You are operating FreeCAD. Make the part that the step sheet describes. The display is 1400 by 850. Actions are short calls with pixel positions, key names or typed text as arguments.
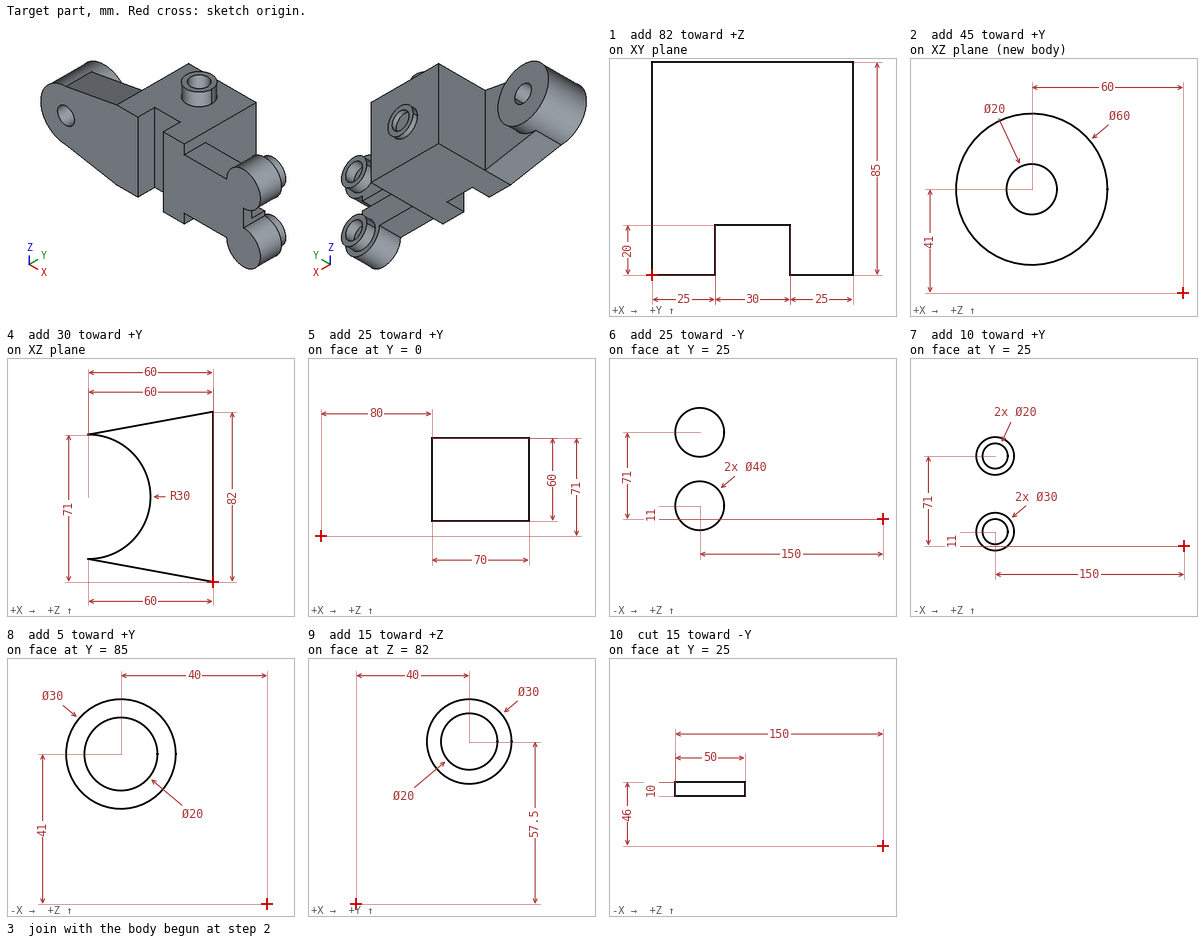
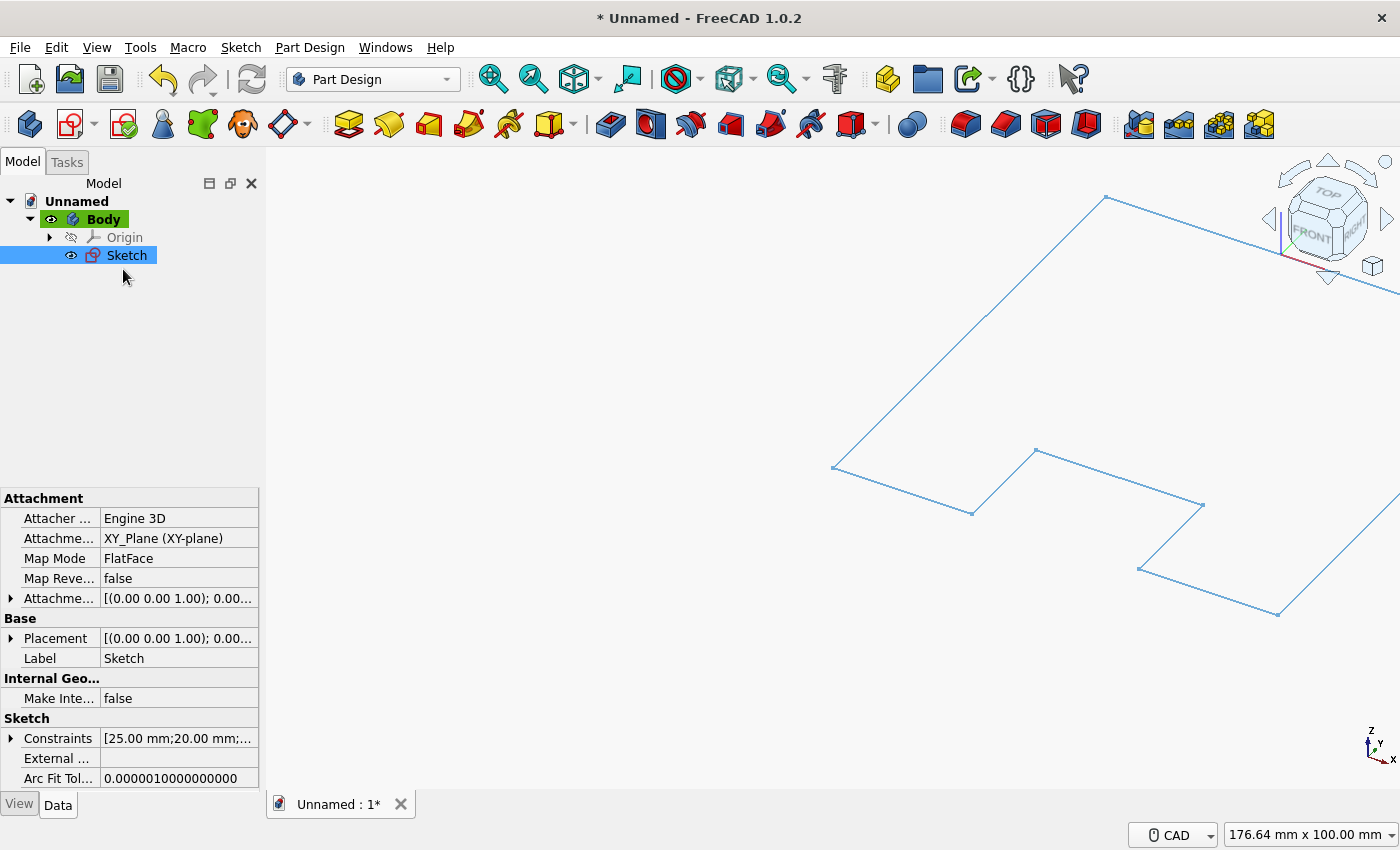
click(350, 124)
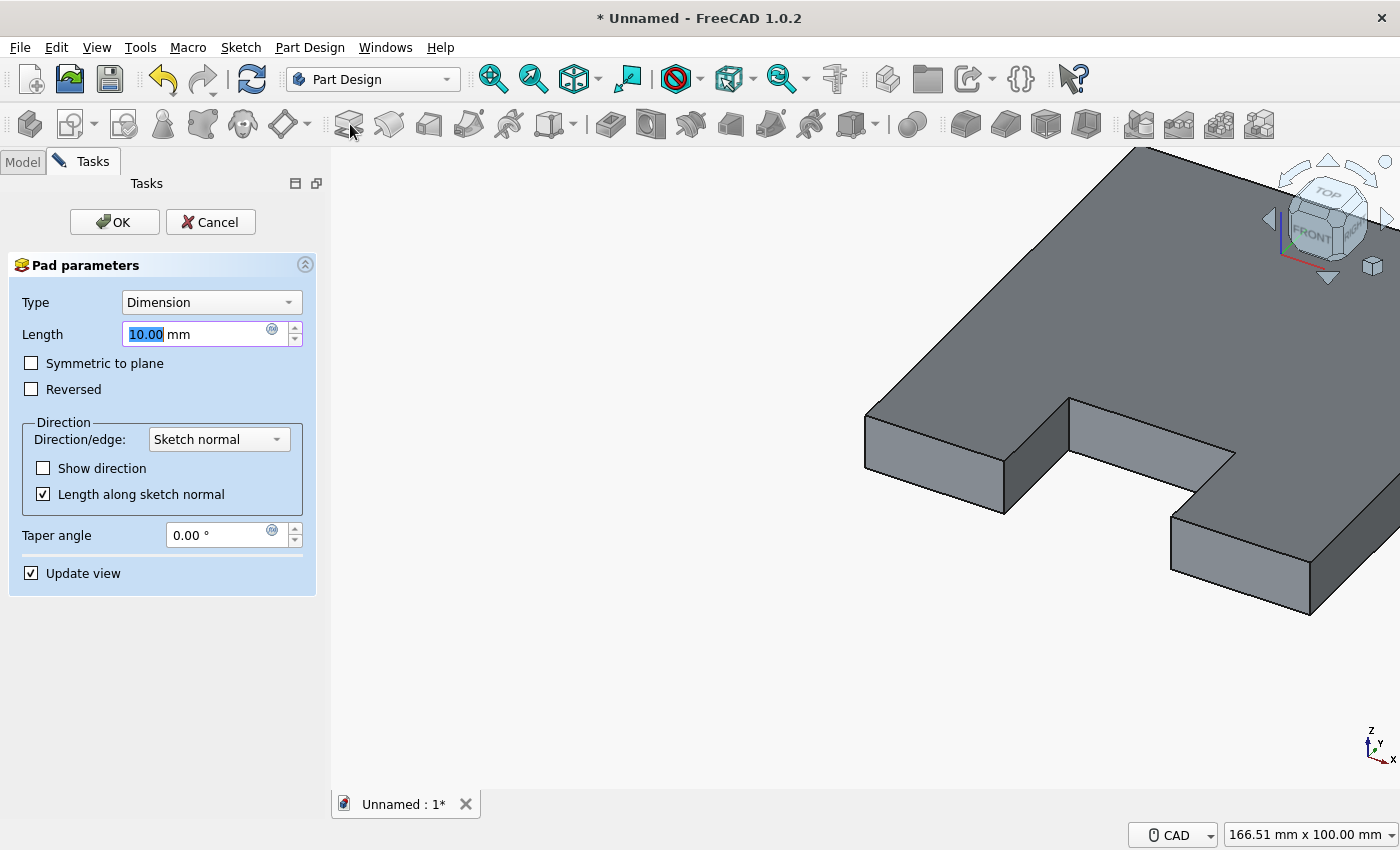
text(82)
key(Tab)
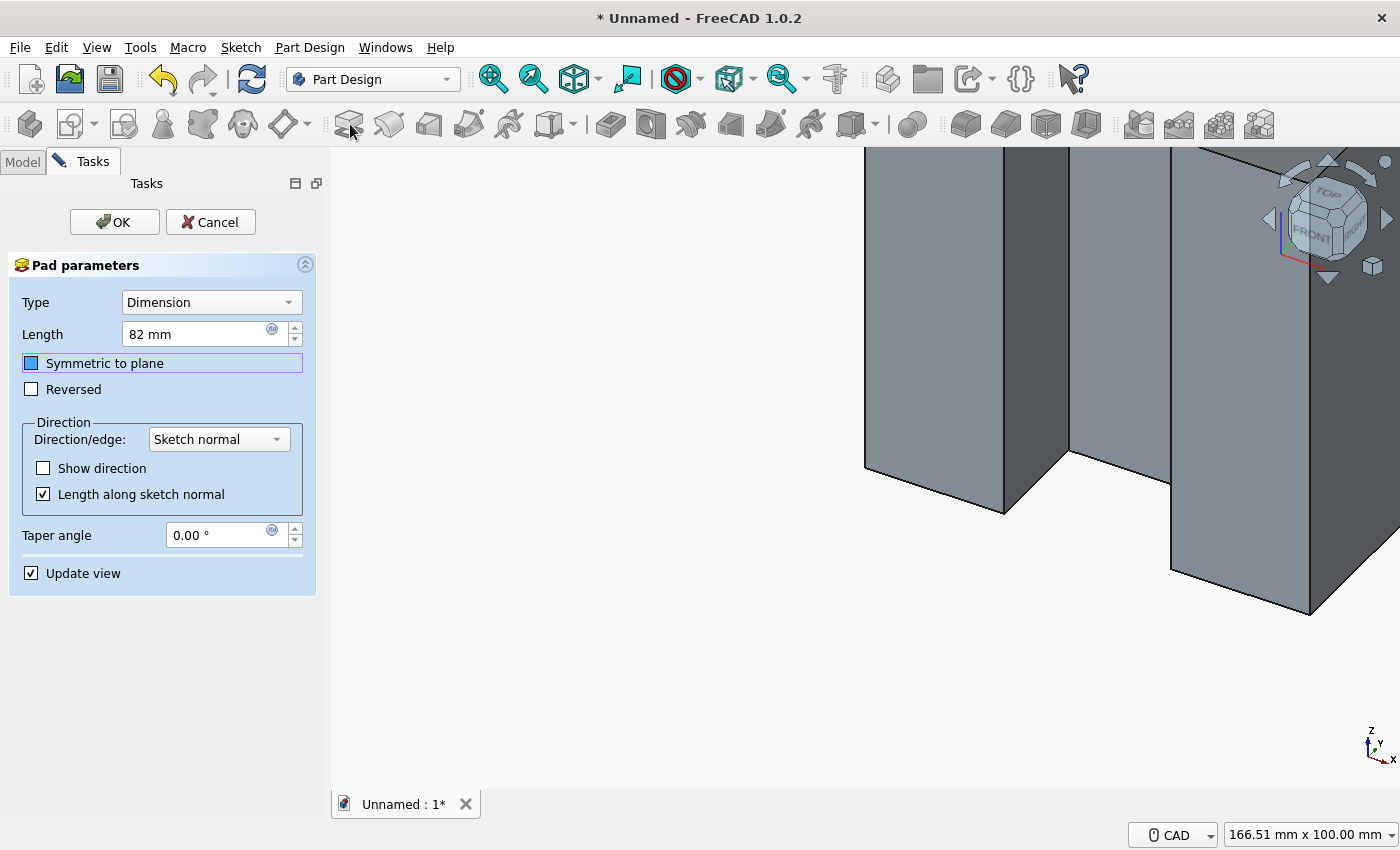
click(115, 222)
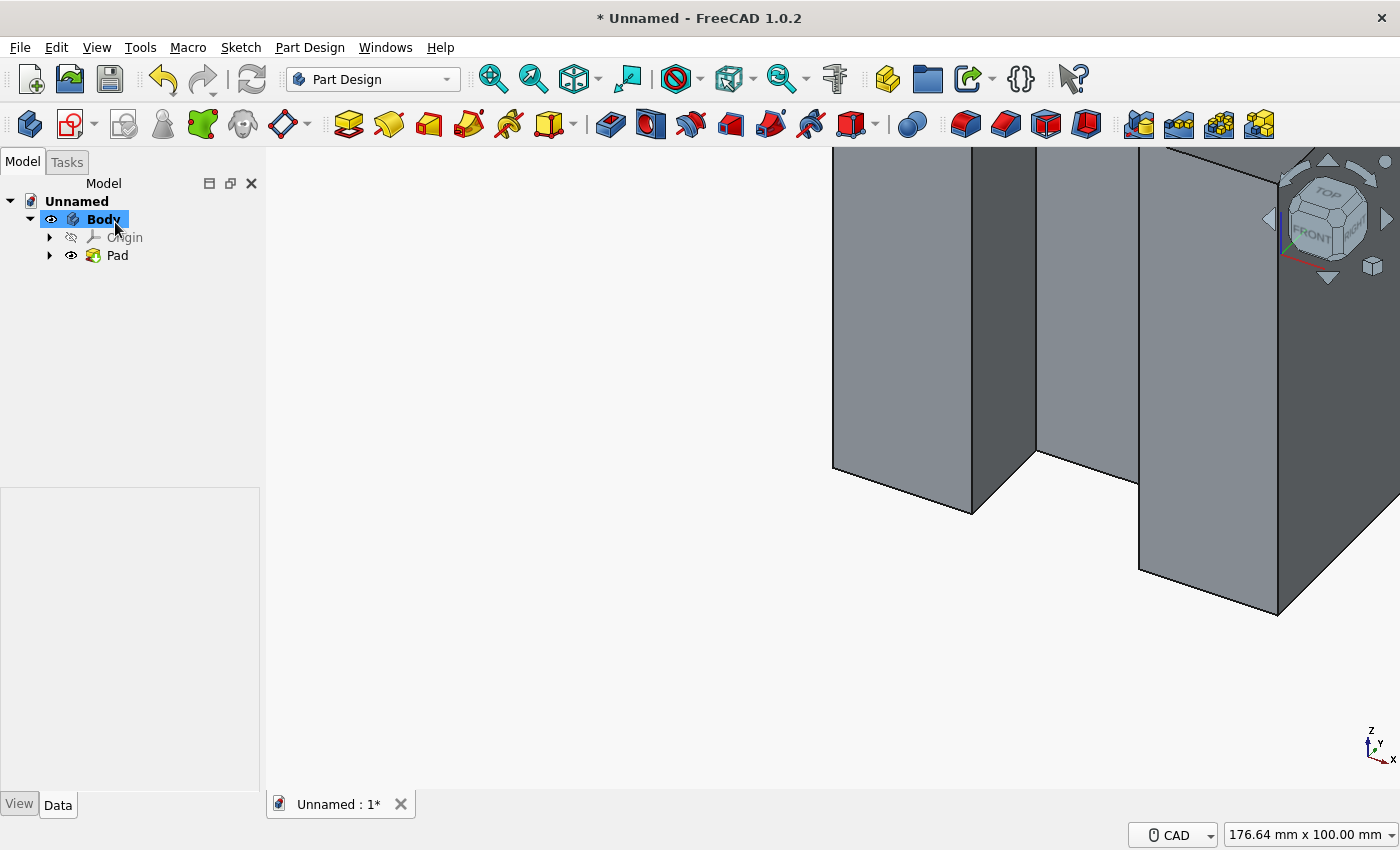
key(v)
key(f)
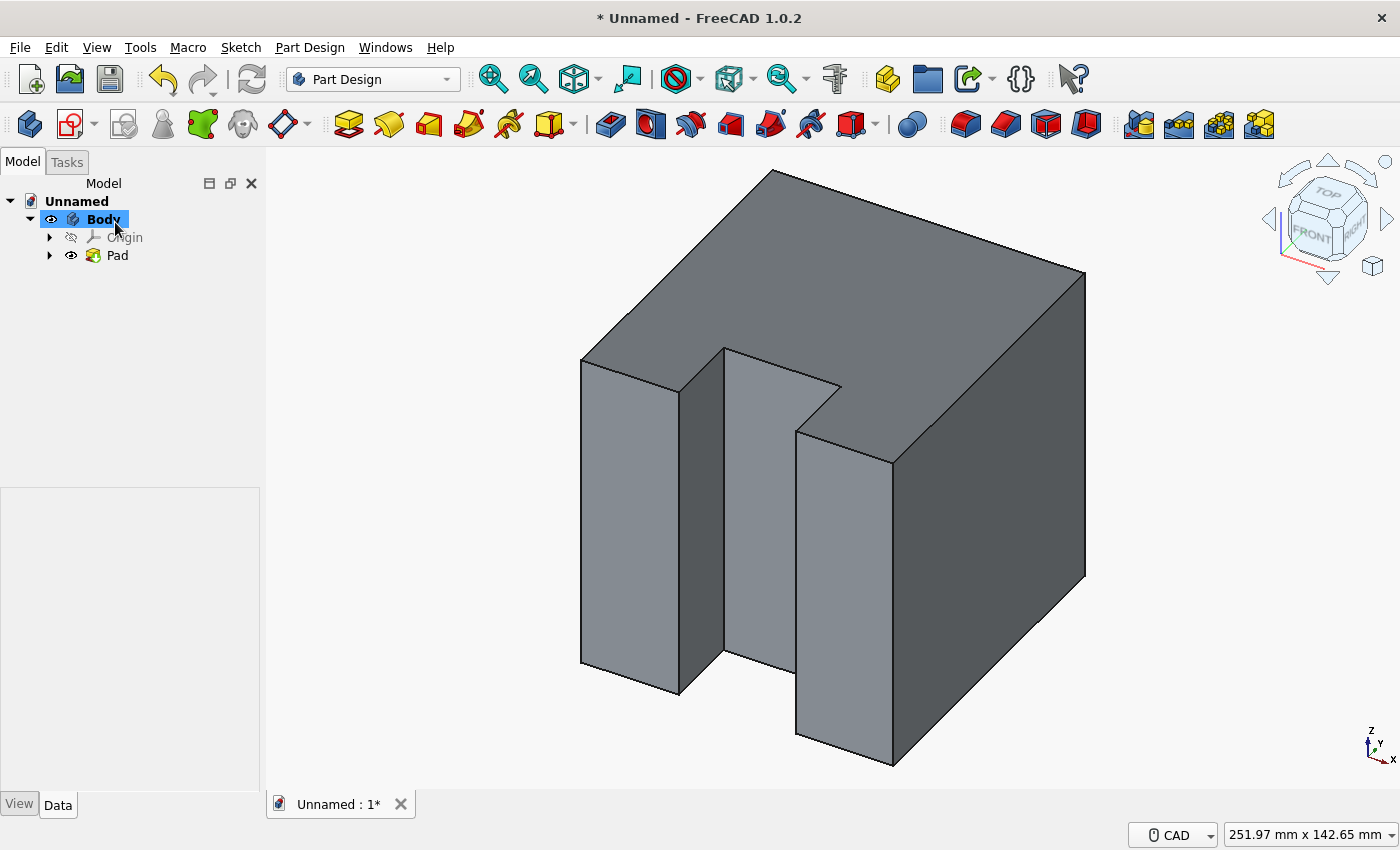
click(30, 124)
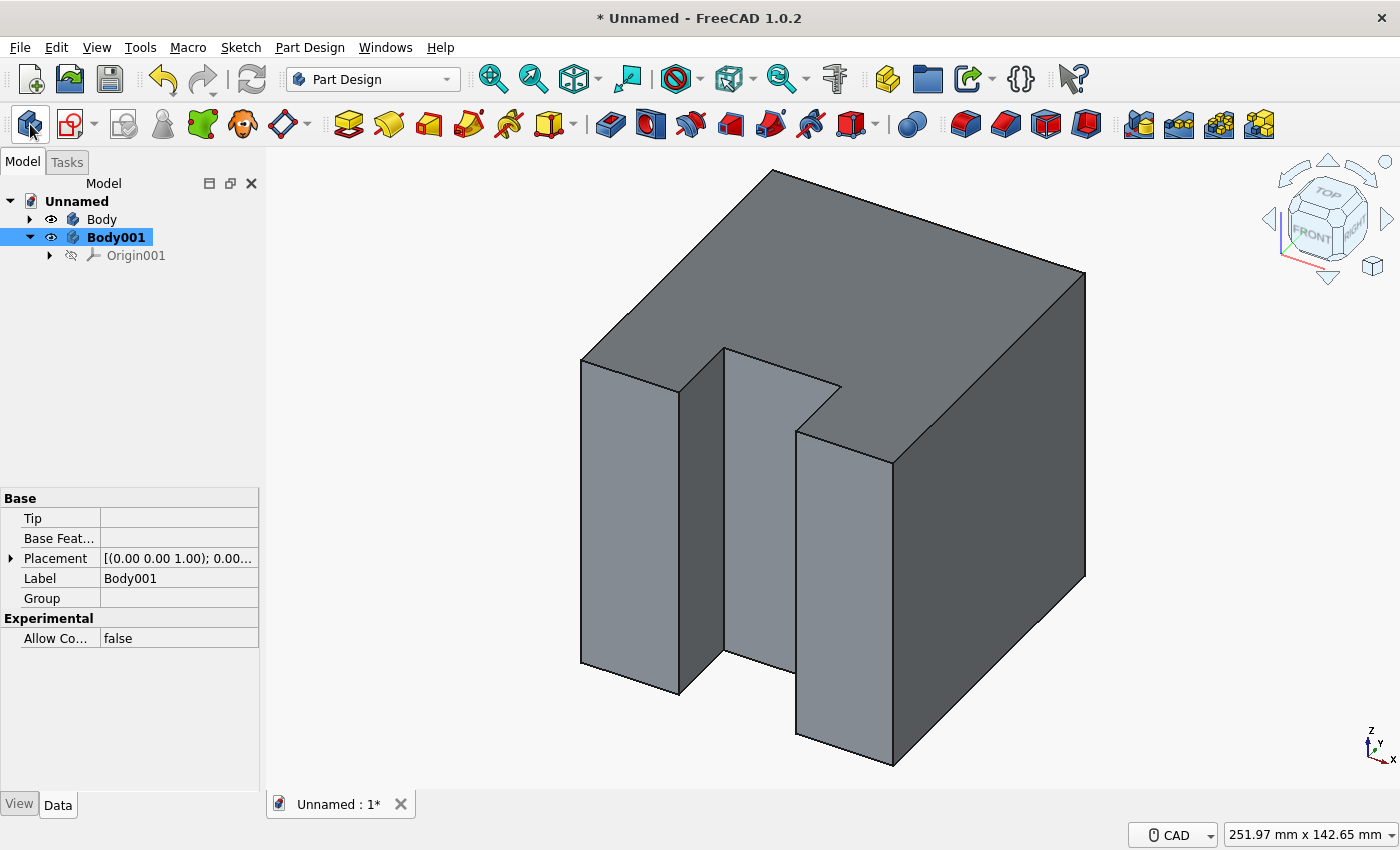
click(306, 749)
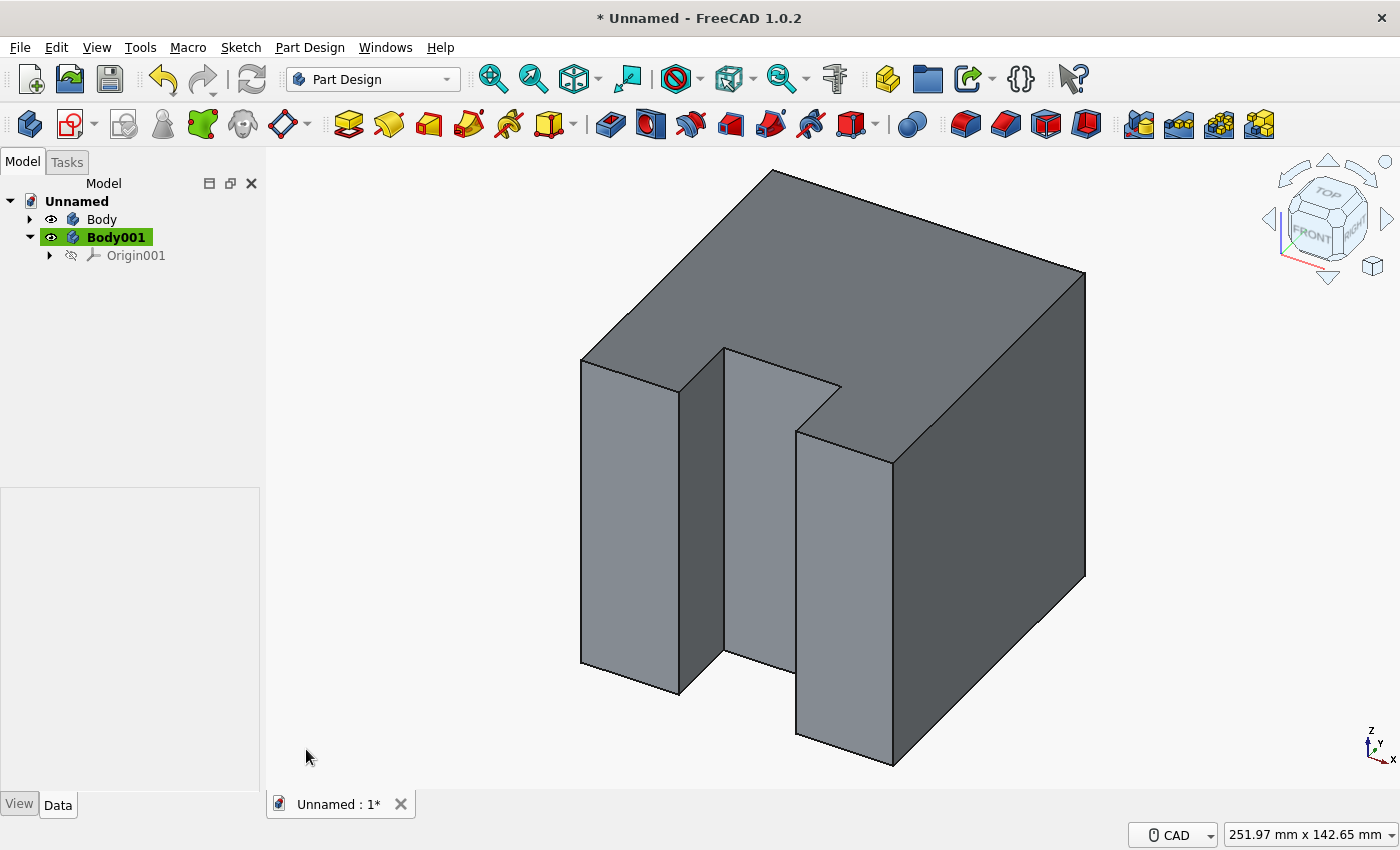
click(70, 124)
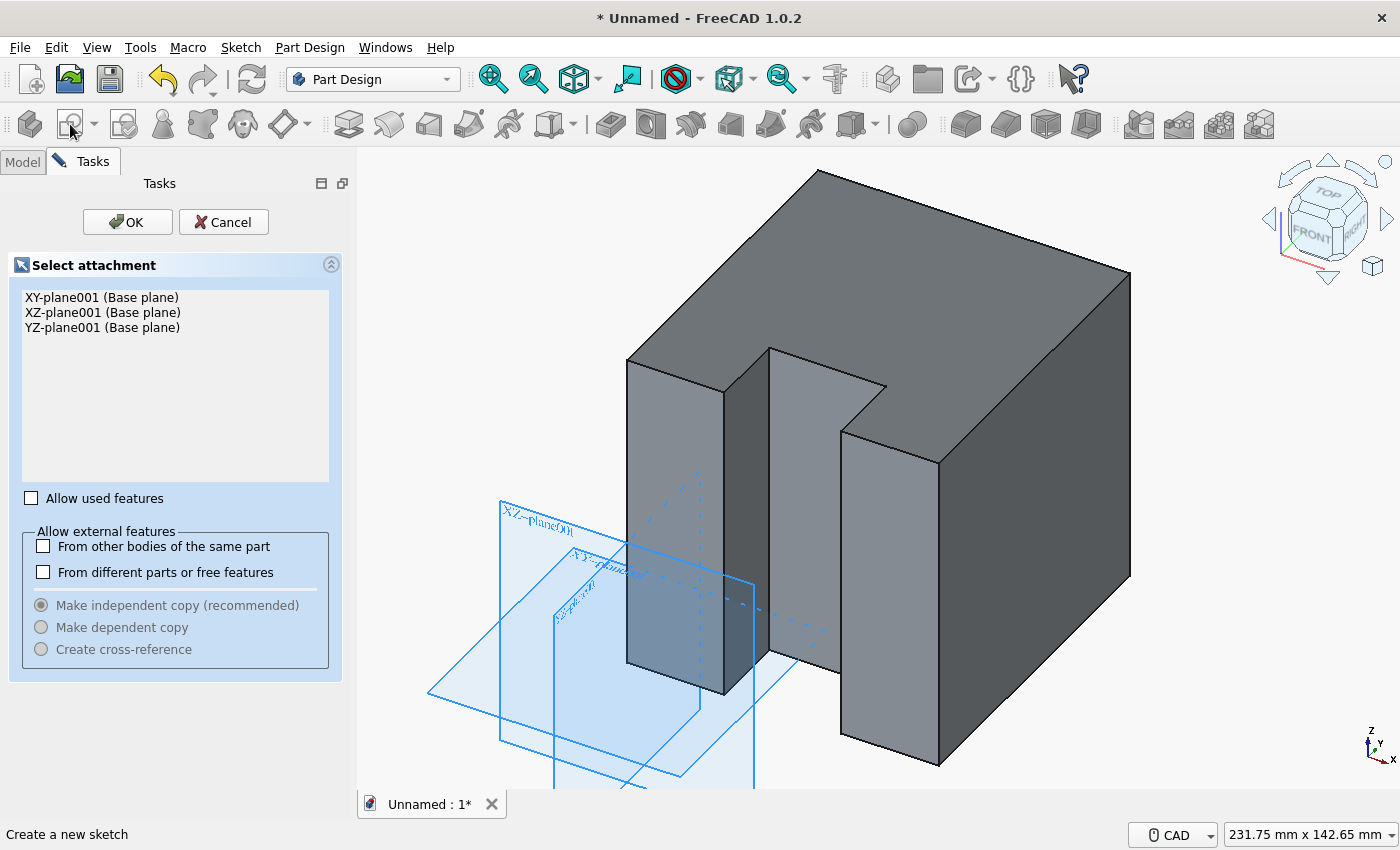
click(82, 312)